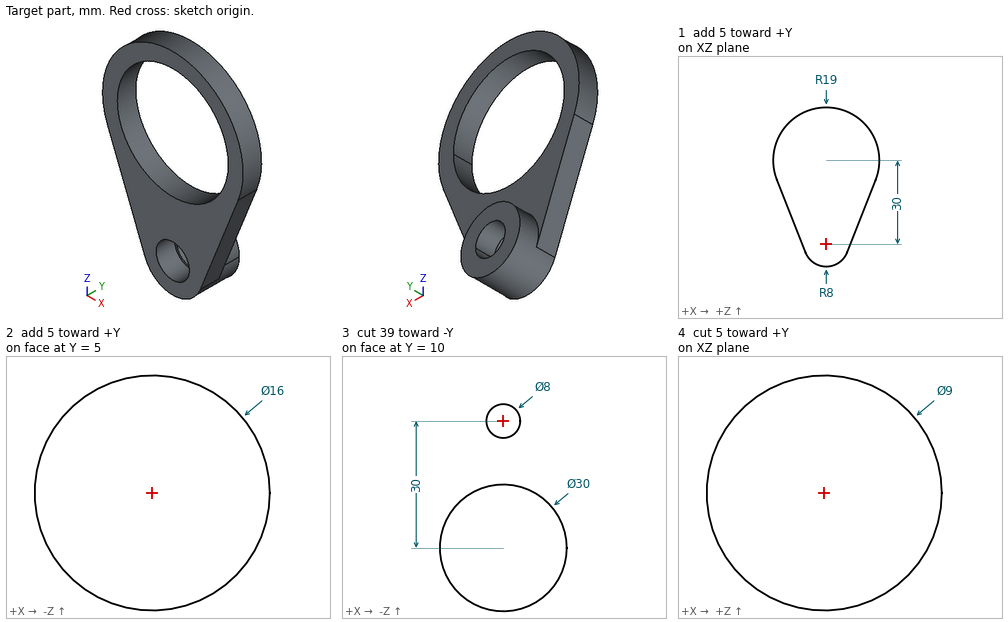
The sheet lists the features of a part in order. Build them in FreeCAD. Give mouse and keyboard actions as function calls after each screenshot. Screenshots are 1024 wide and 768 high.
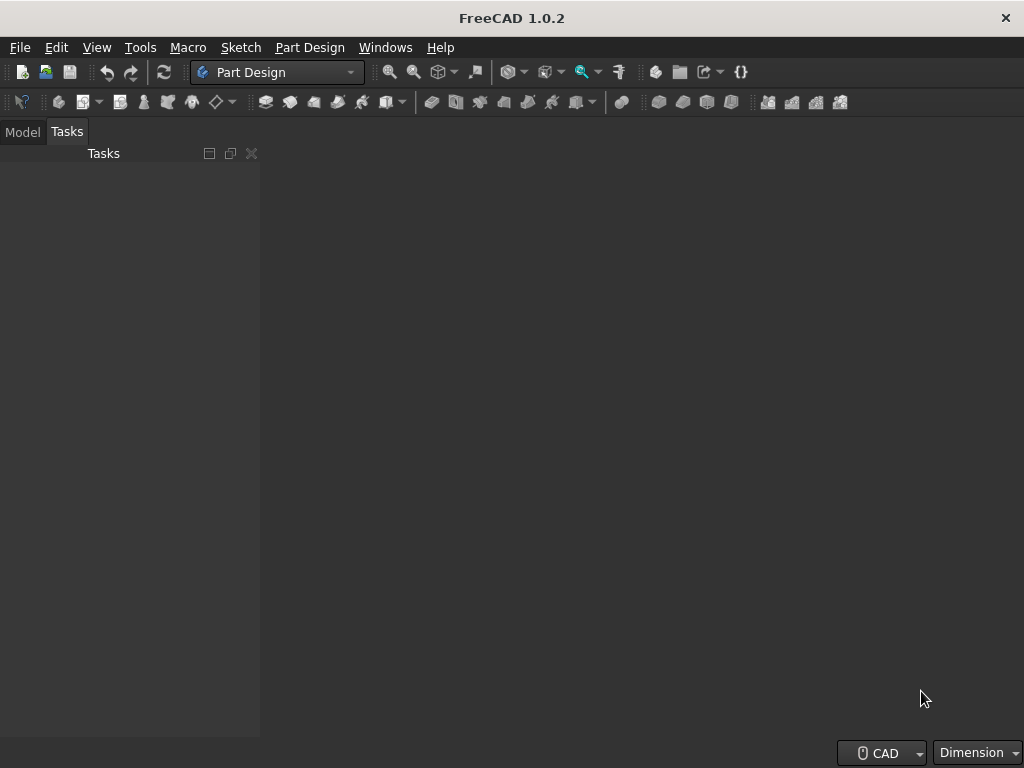
click(22, 72)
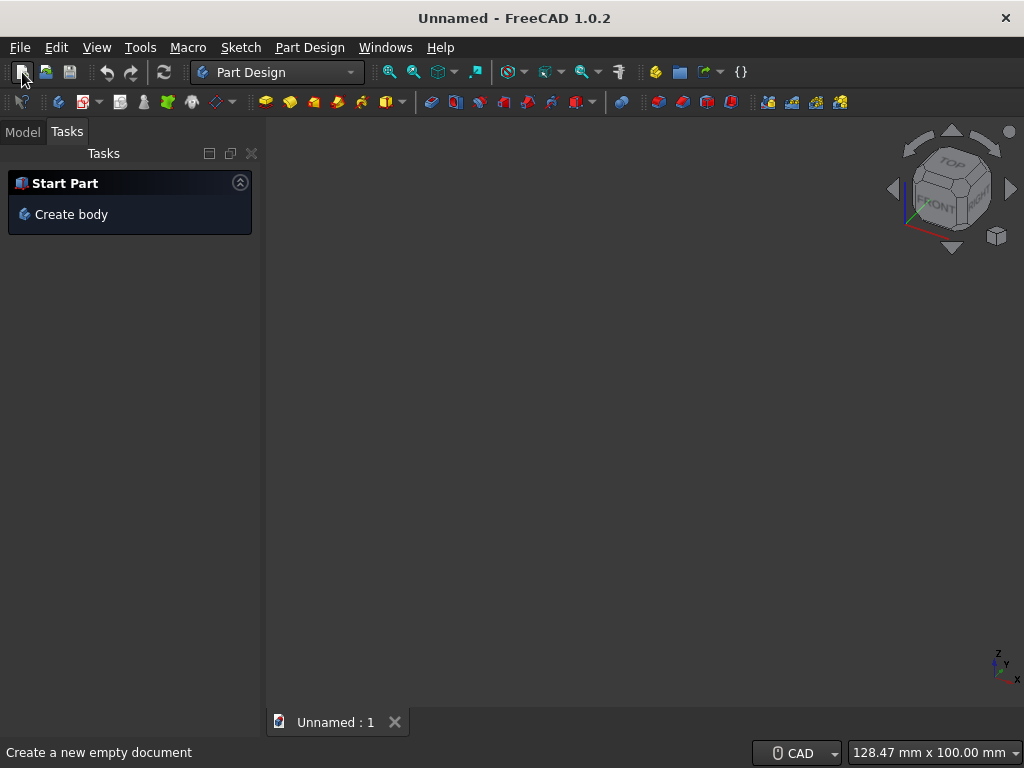
click(84, 102)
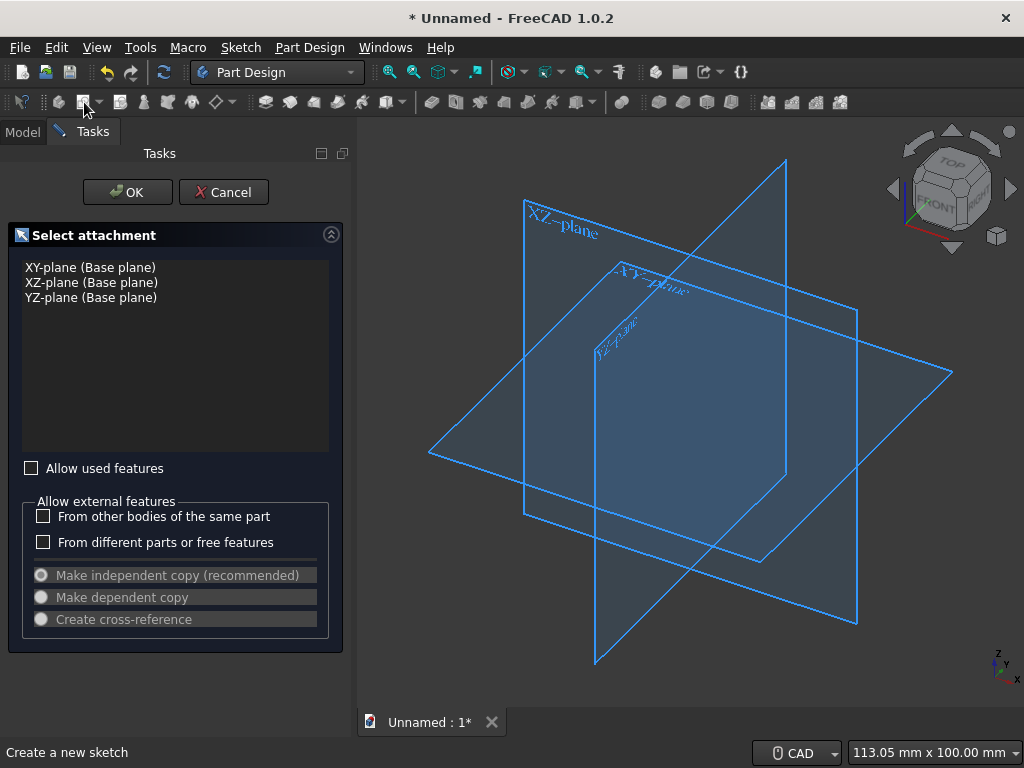
click(82, 282)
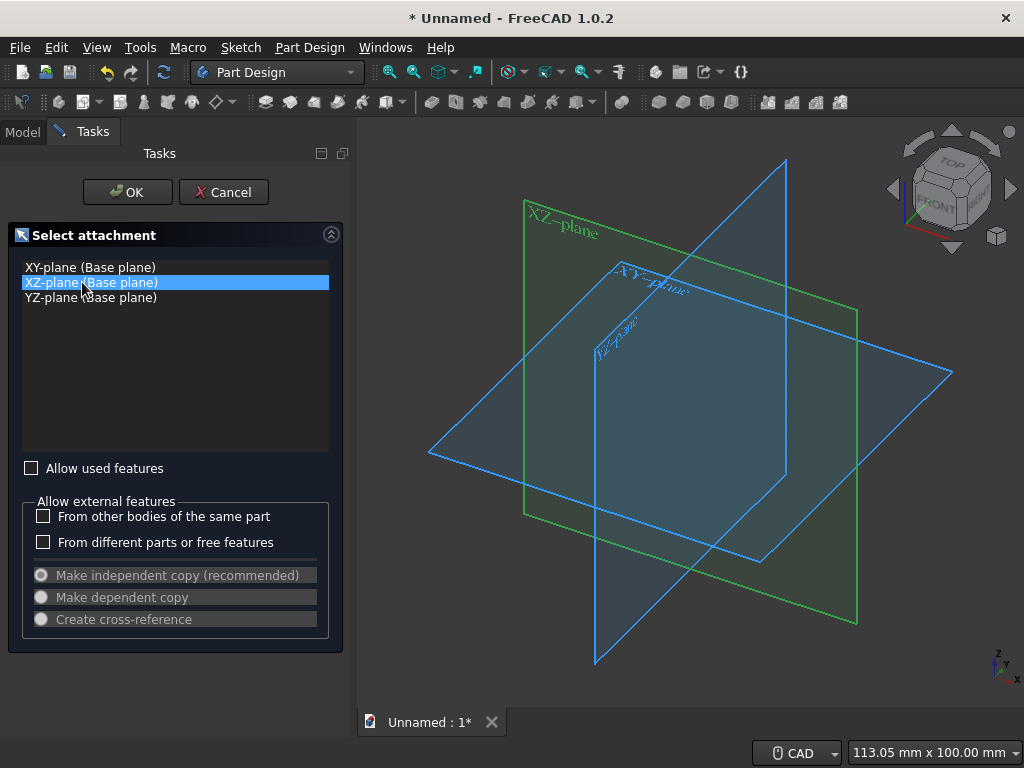
click(128, 192)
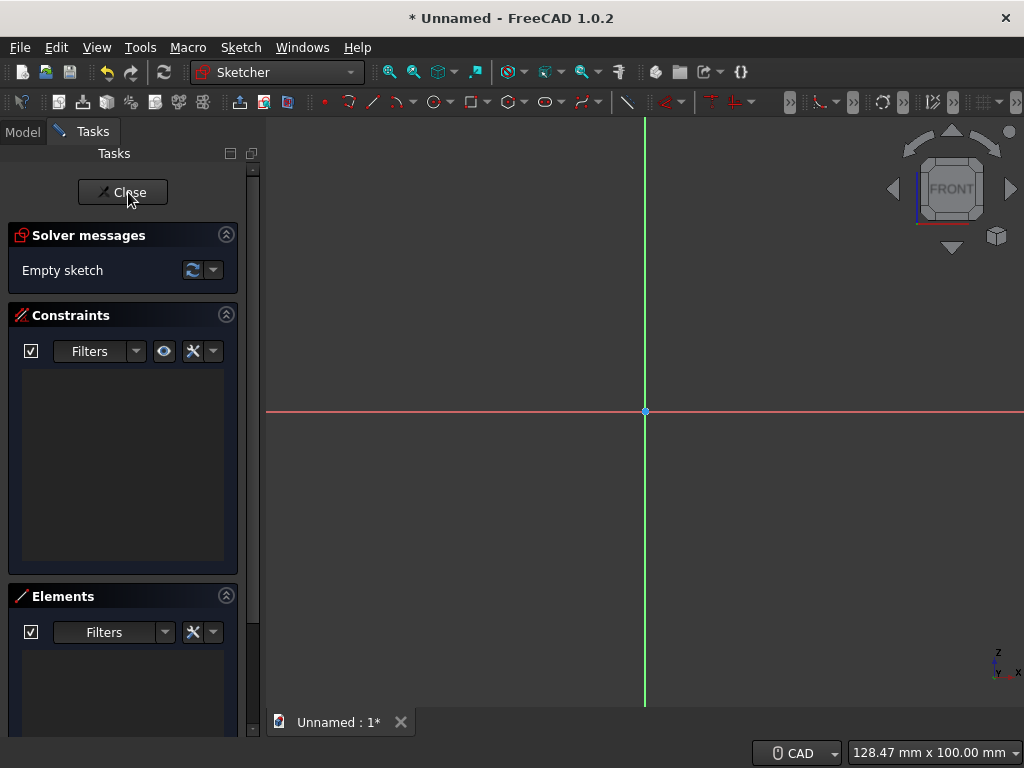
scroll(294, 679, down, 1)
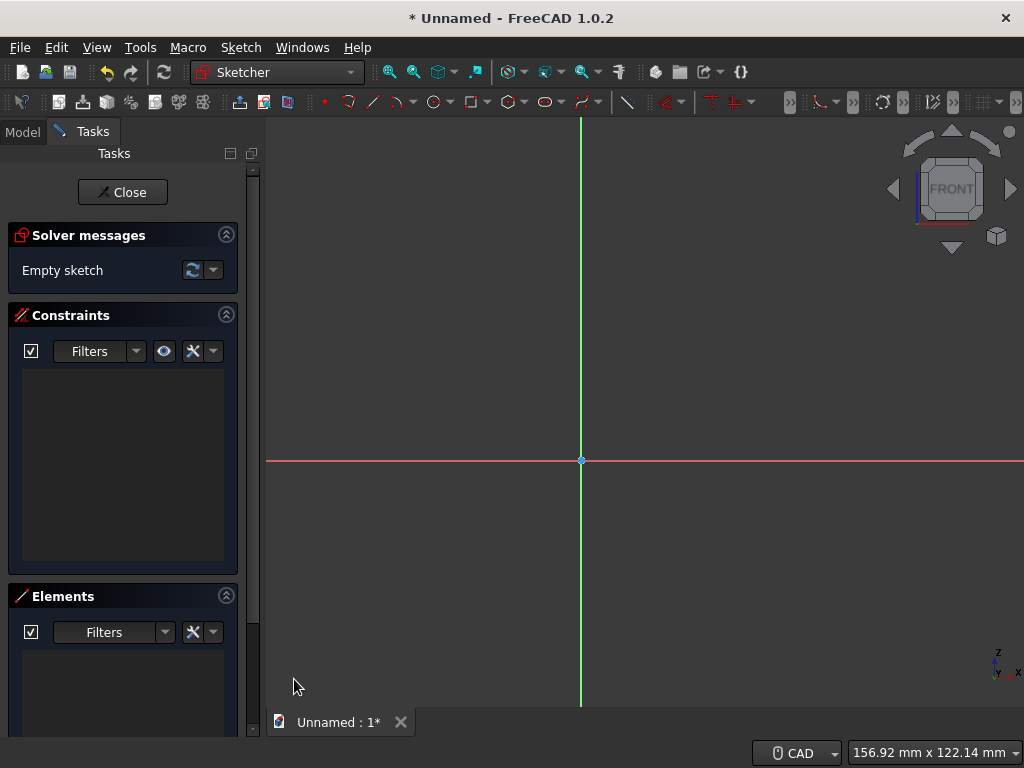
scroll(591, 259, up, 2)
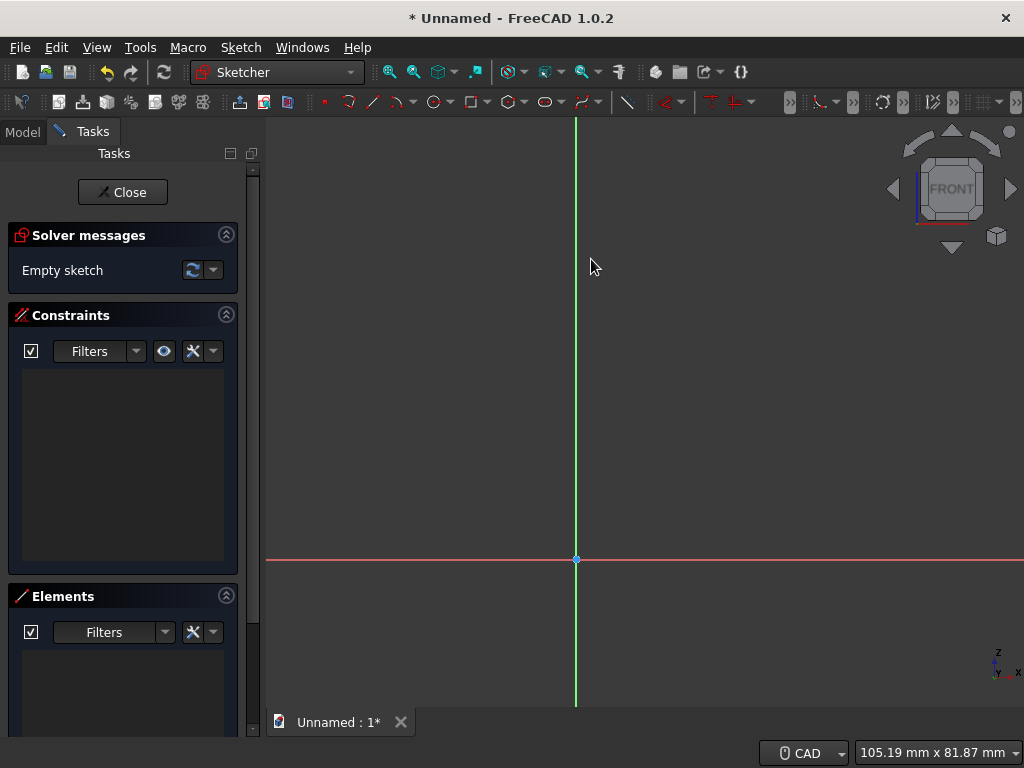
click(374, 102)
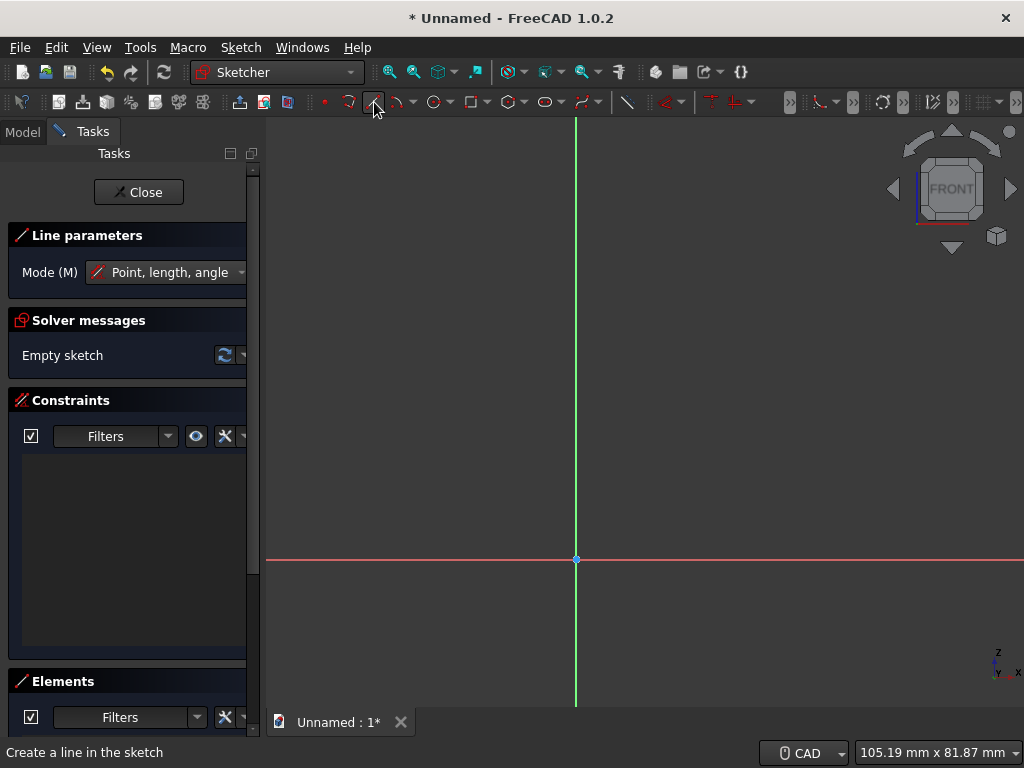
click(523, 581)
click(449, 394)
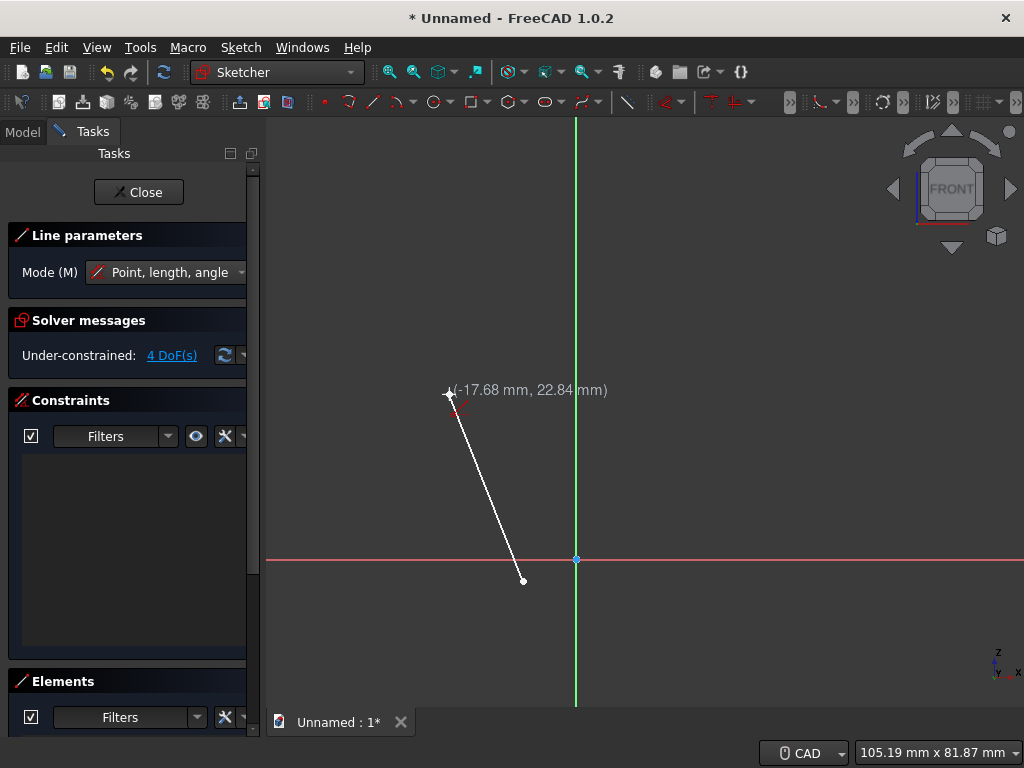
click(704, 394)
click(630, 581)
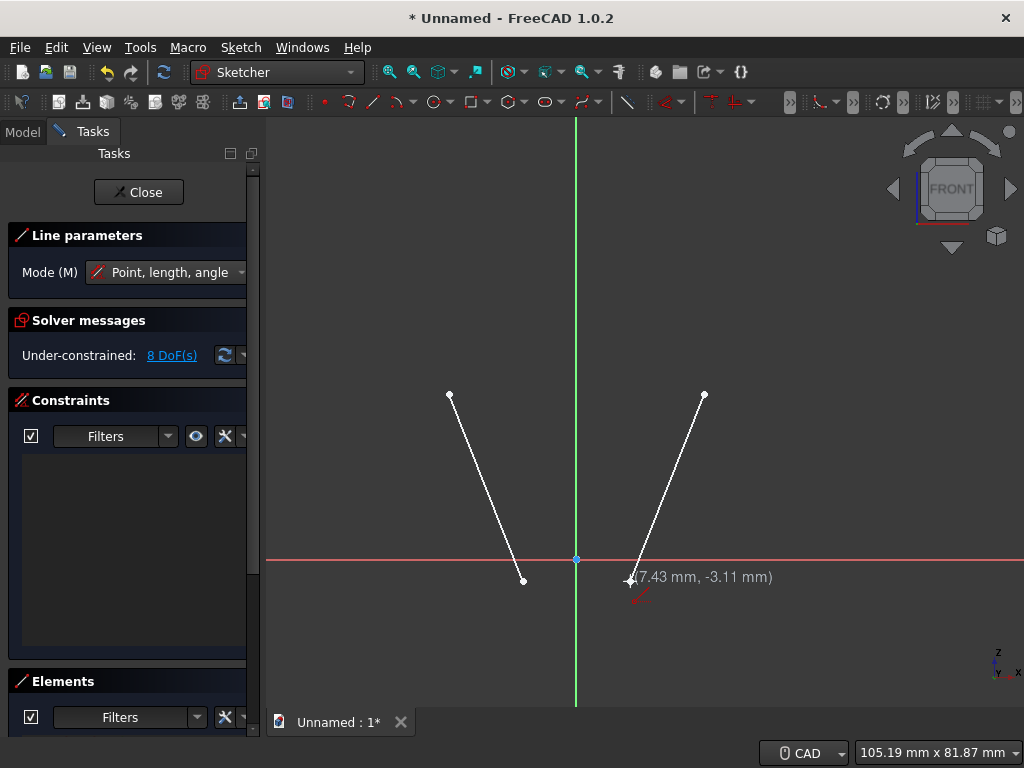
click(416, 102)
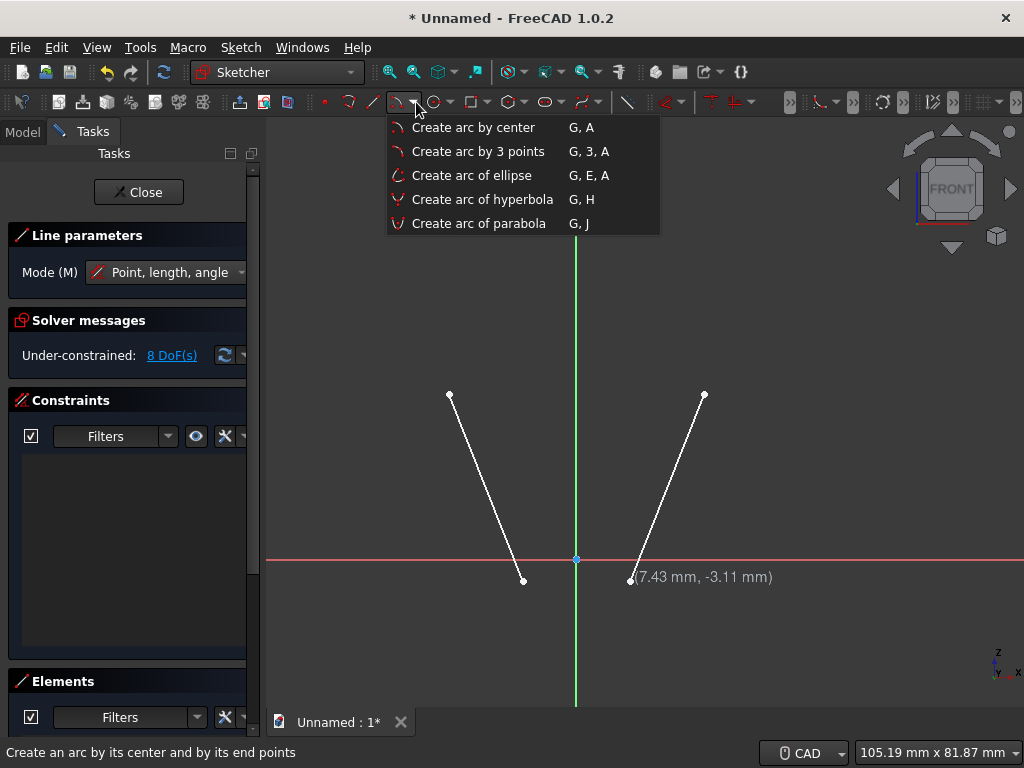
click(524, 151)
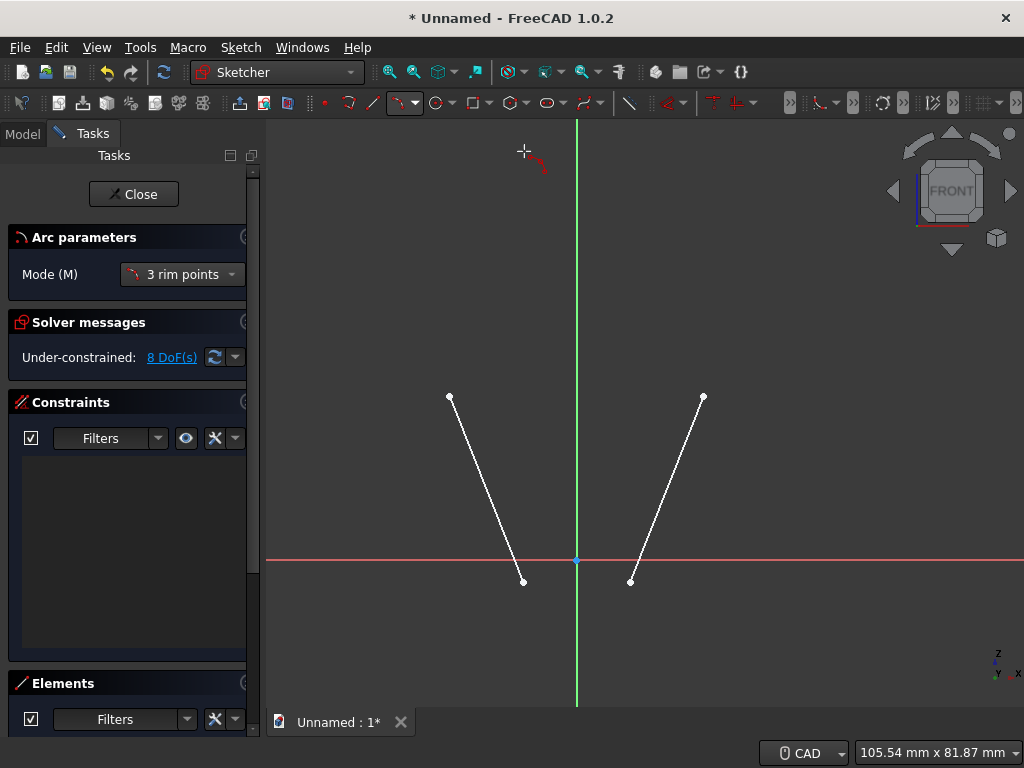
click(450, 396)
click(704, 396)
click(628, 218)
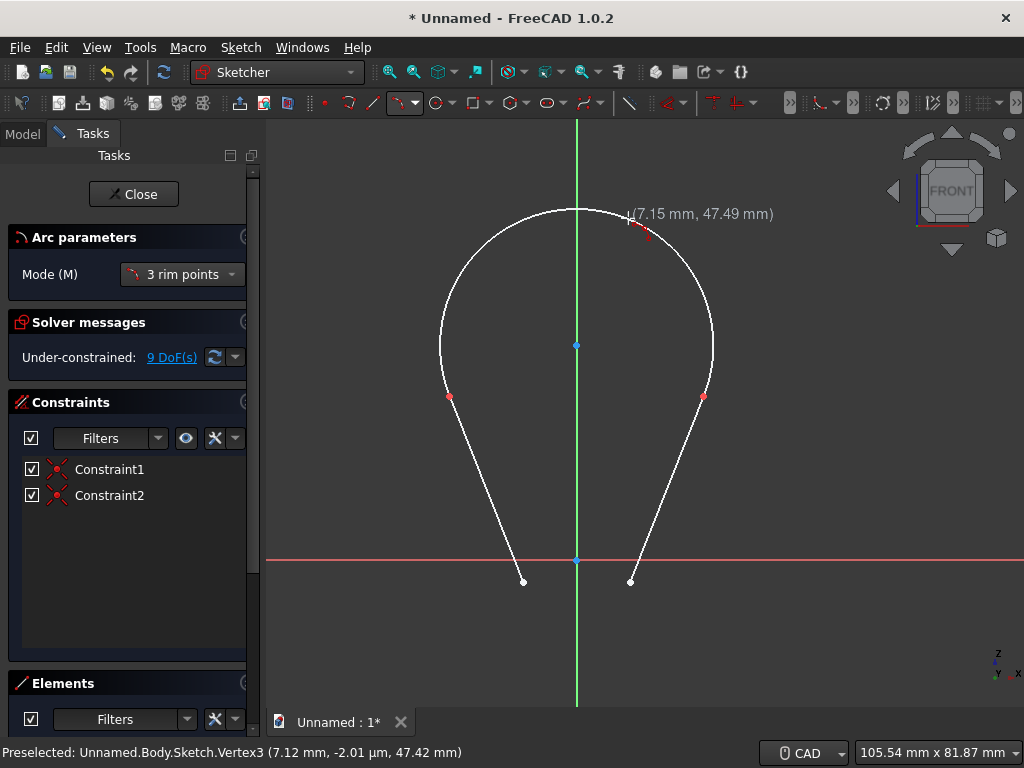
click(630, 582)
click(523, 582)
click(550, 611)
key(Escape)